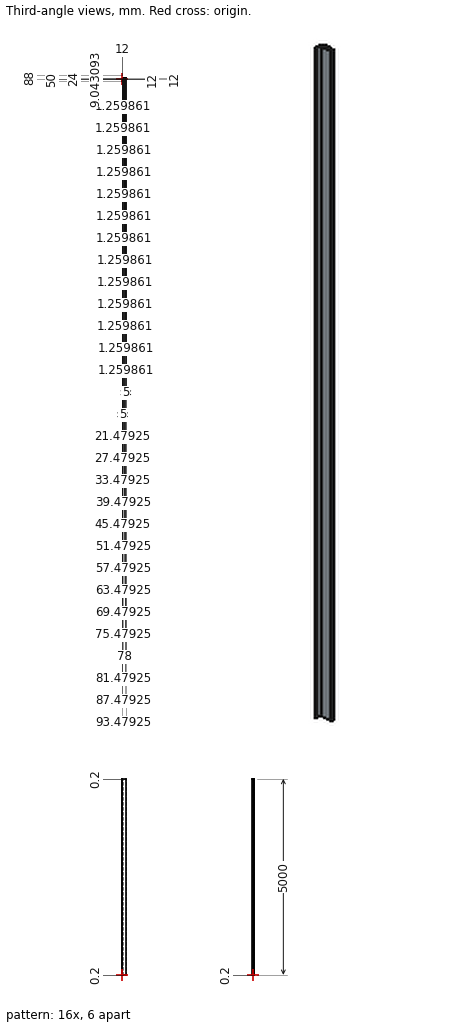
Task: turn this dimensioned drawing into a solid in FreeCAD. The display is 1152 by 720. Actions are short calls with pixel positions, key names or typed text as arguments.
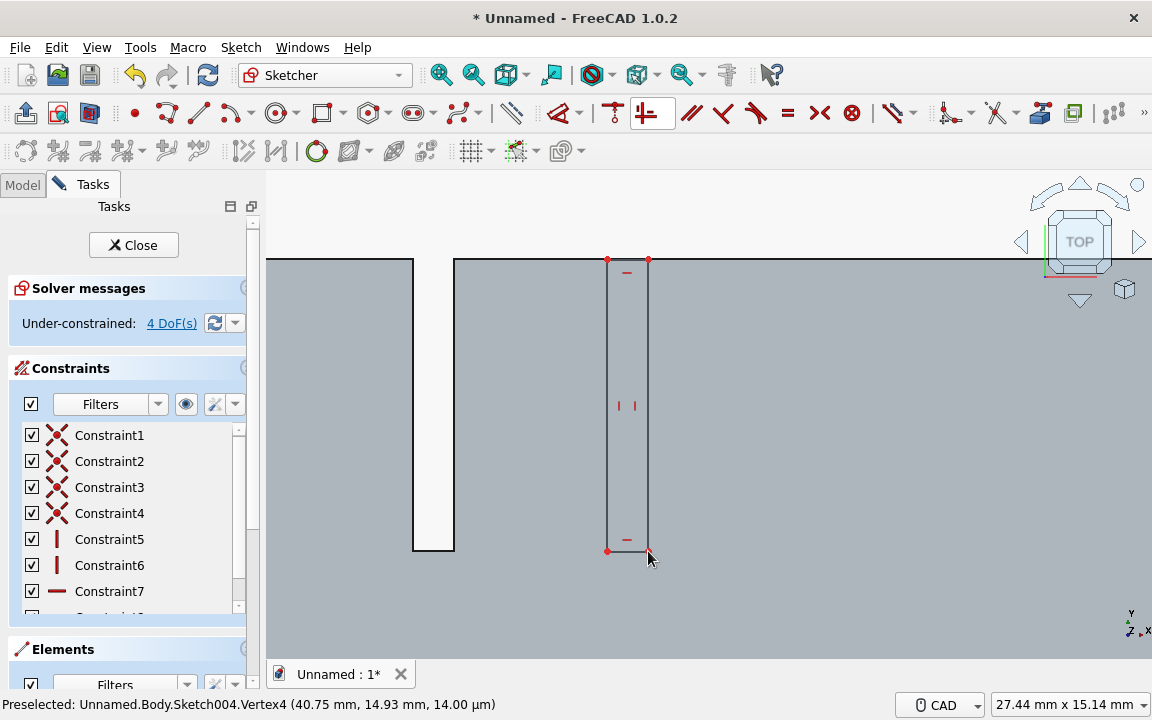
click(558, 114)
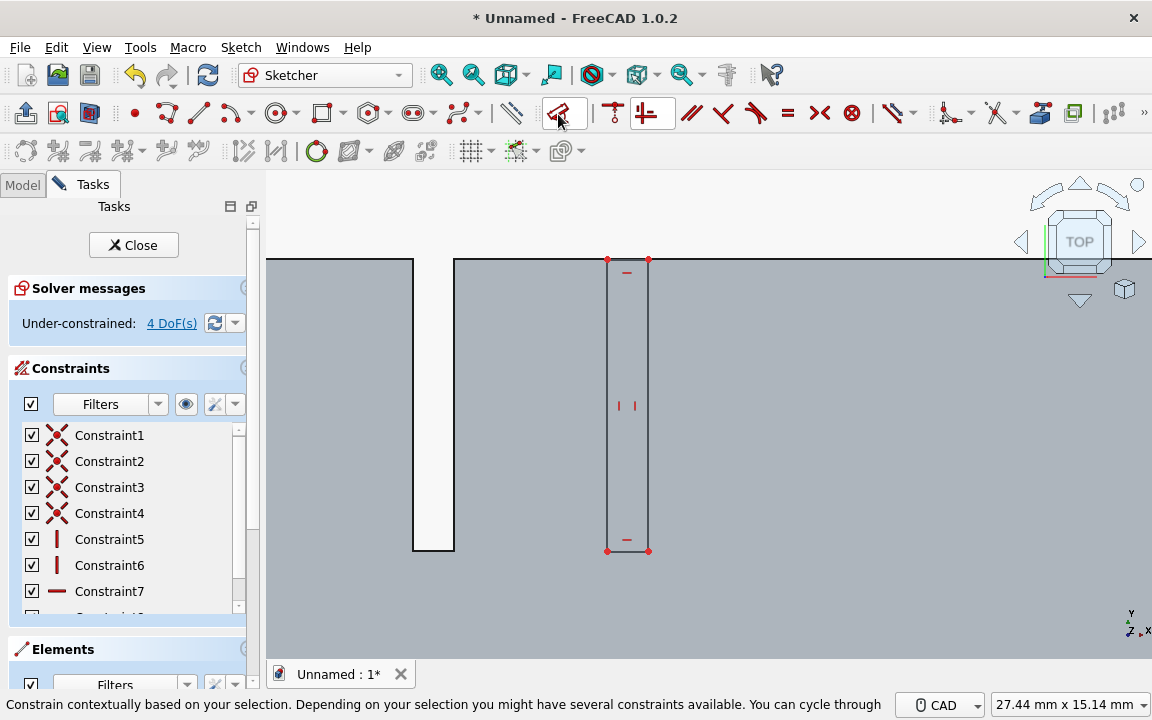
click(607, 260)
click(641, 575)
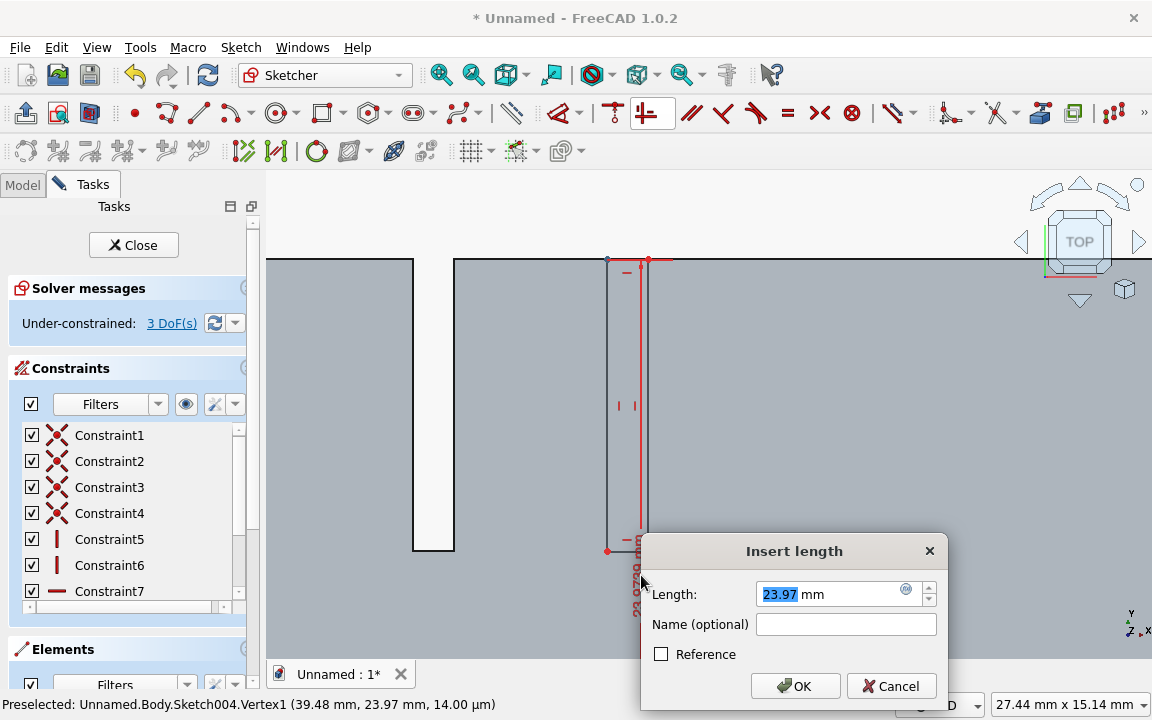
text(24)
key(Return)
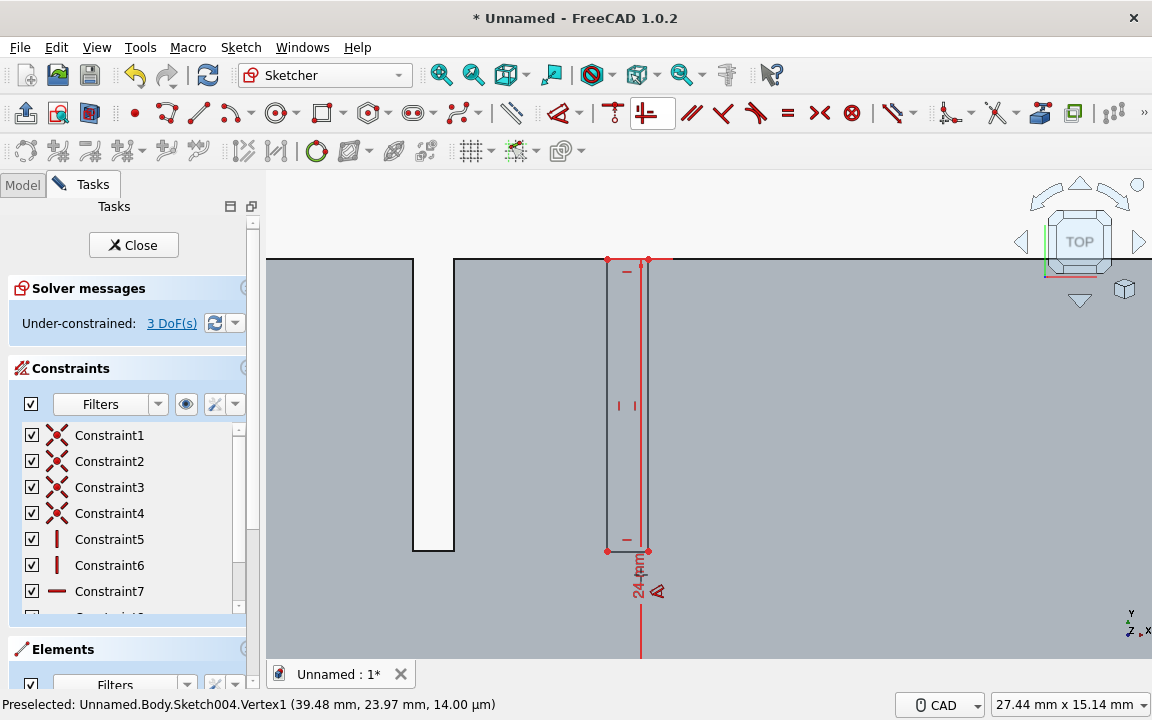
click(607, 347)
click(573, 406)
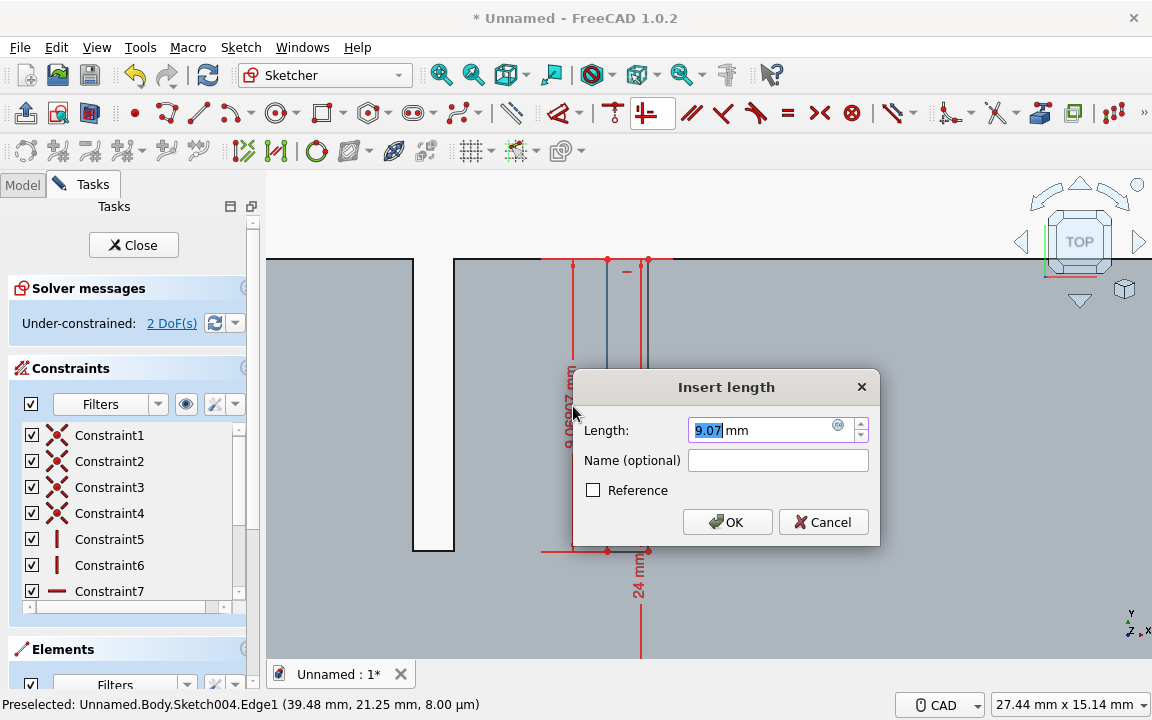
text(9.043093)
key(Return)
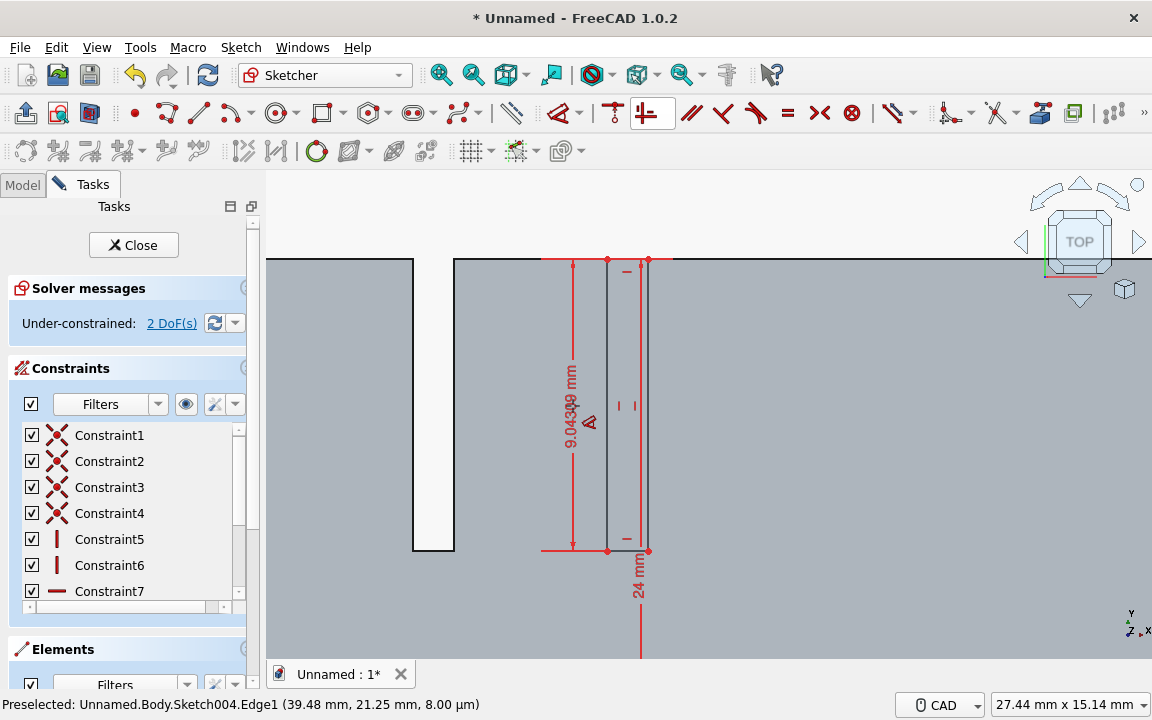
click(619, 551)
click(628, 517)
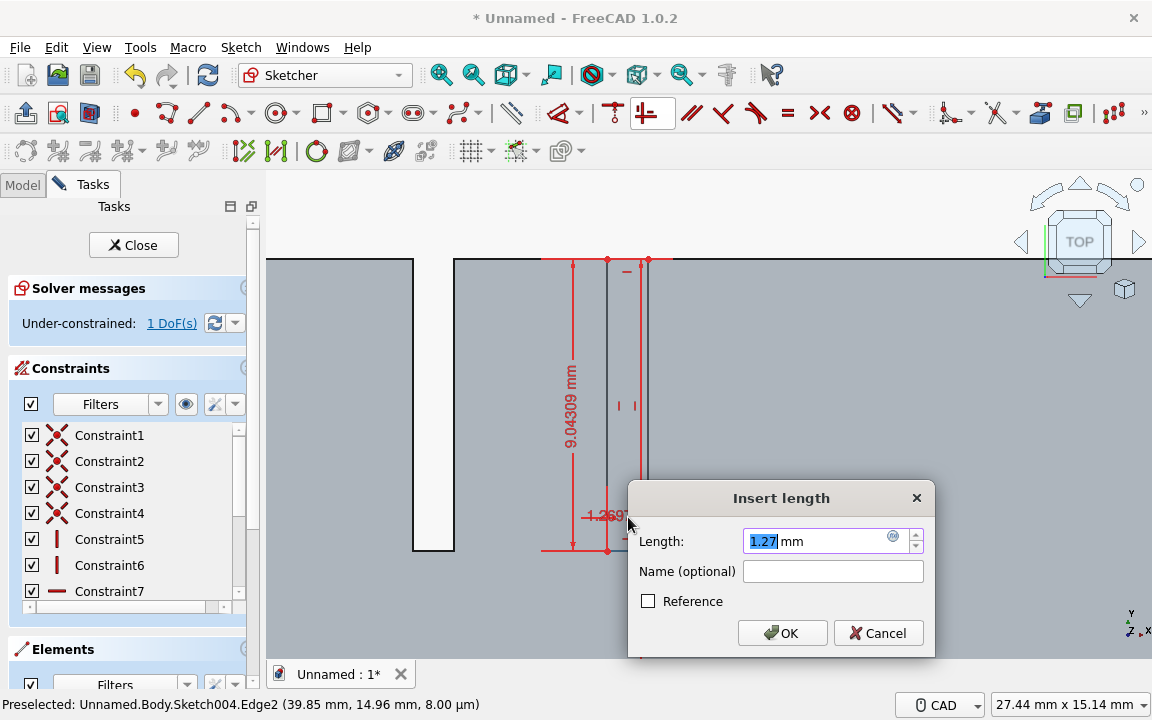
text(1.259861)
key(Return)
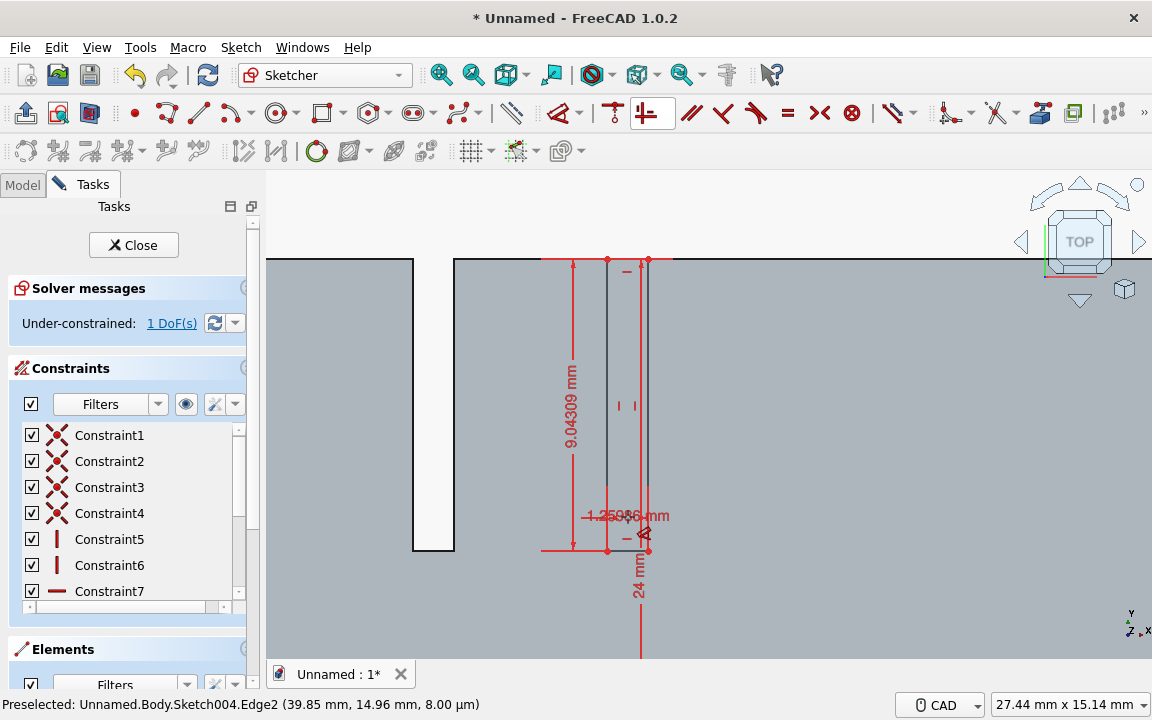
click(607, 259)
click(451, 225)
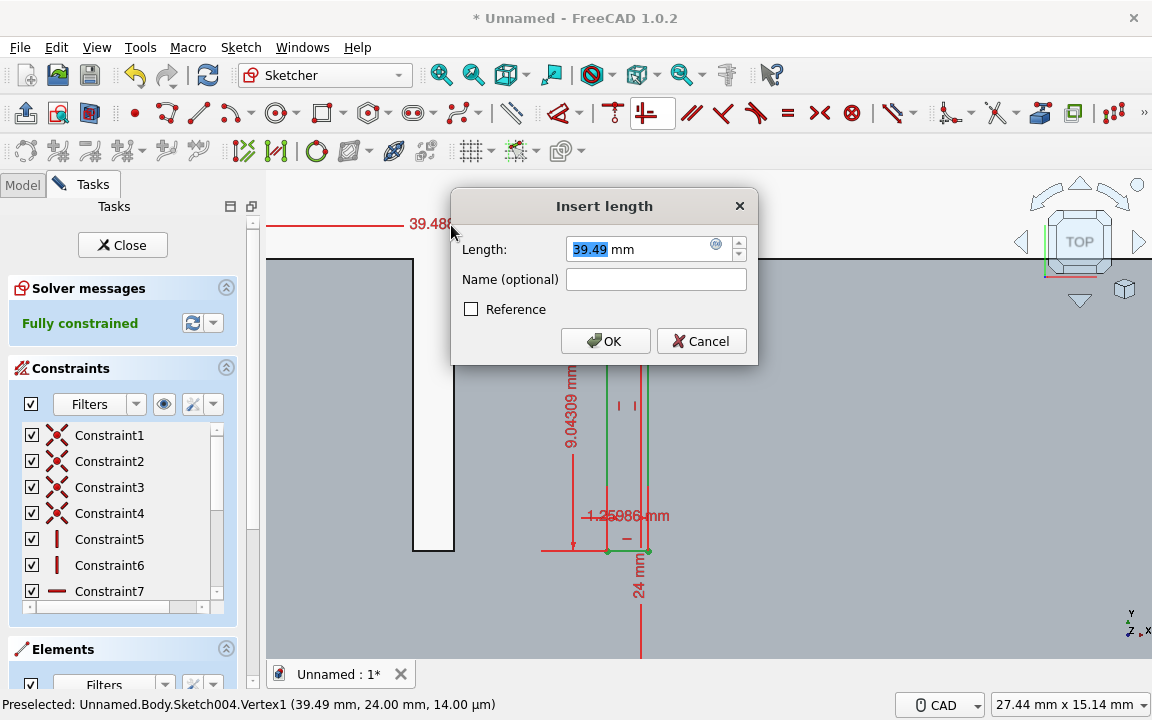
text(39.47925)
key(Return)
key(Escape)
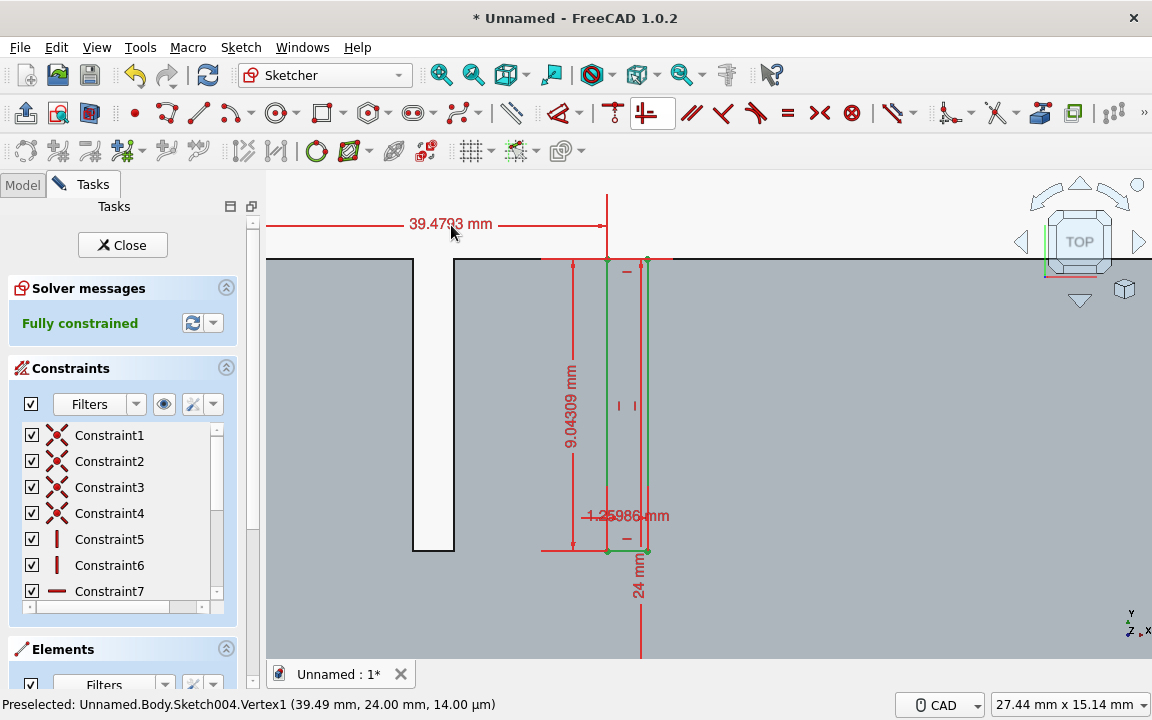
click(123, 245)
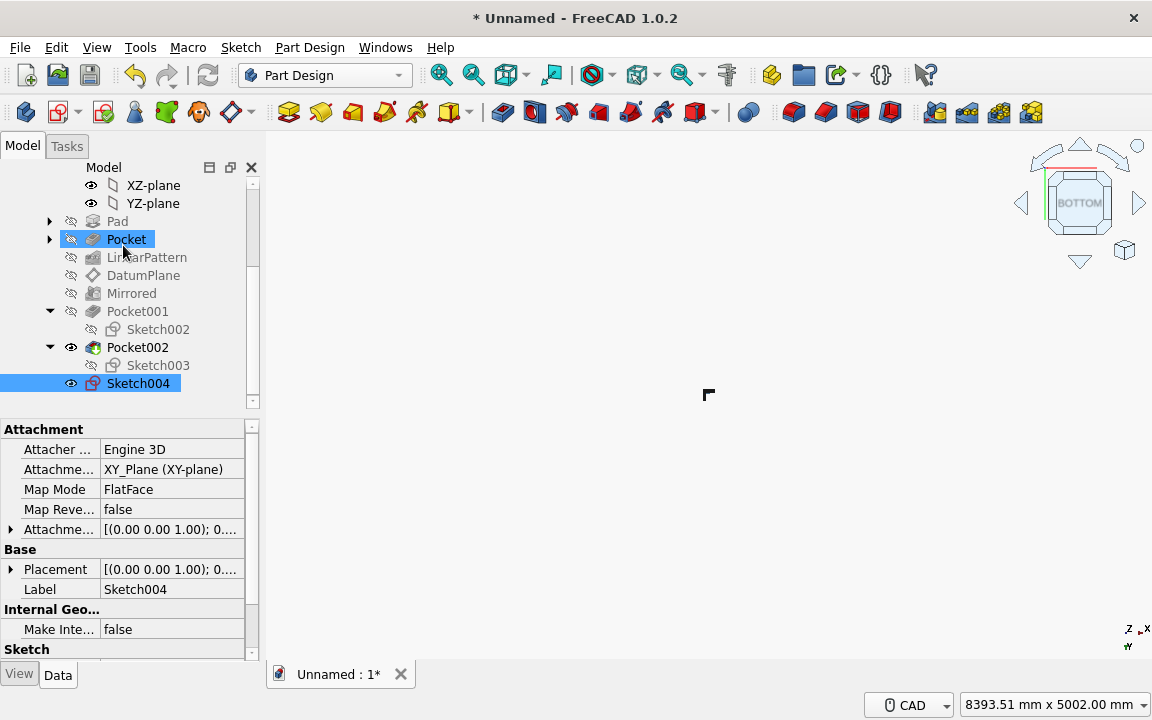
click(504, 112)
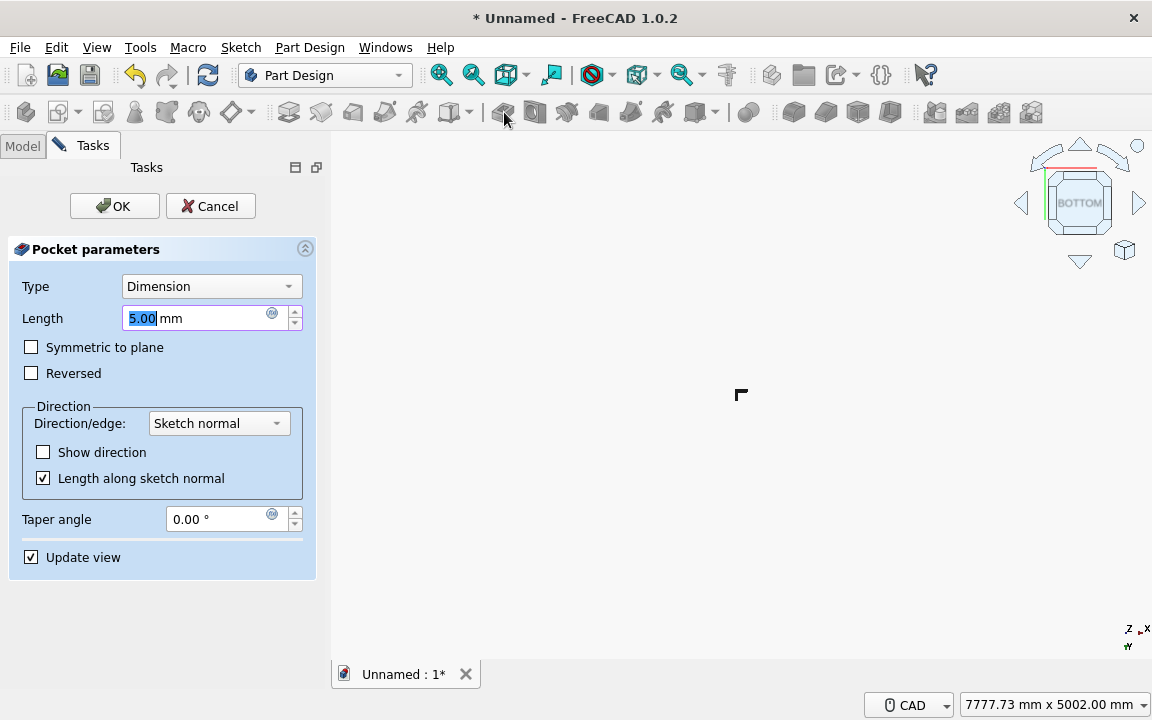
text(0.2)
key(Tab)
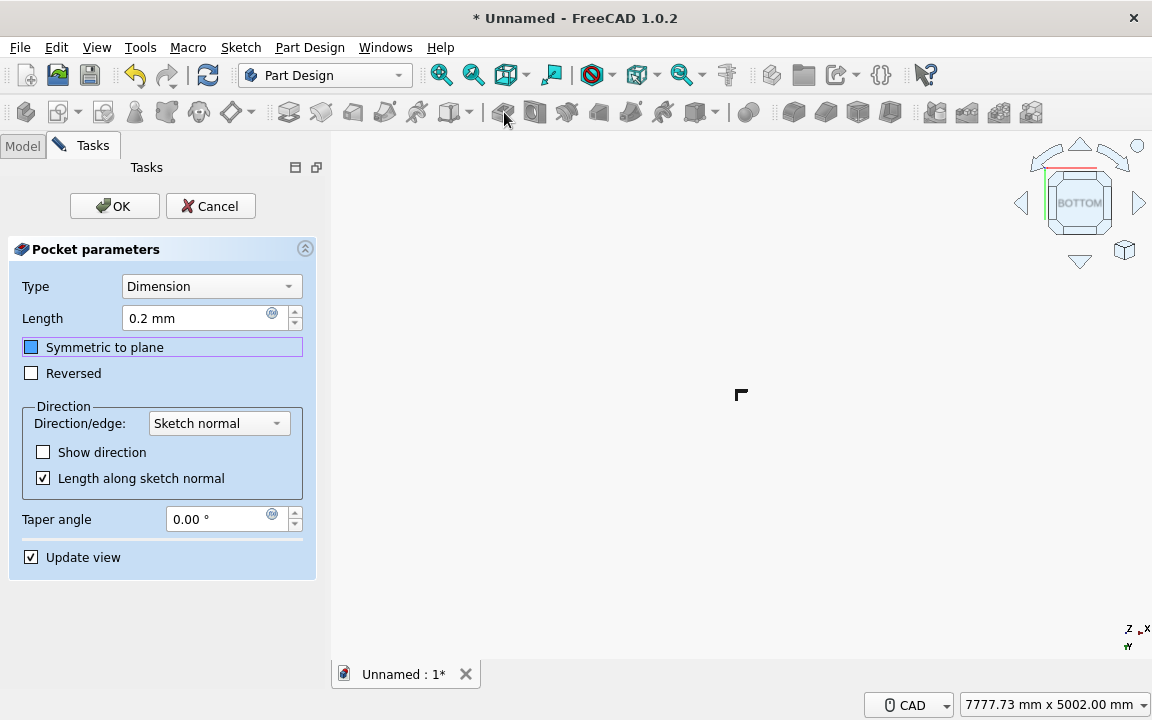
click(30, 373)